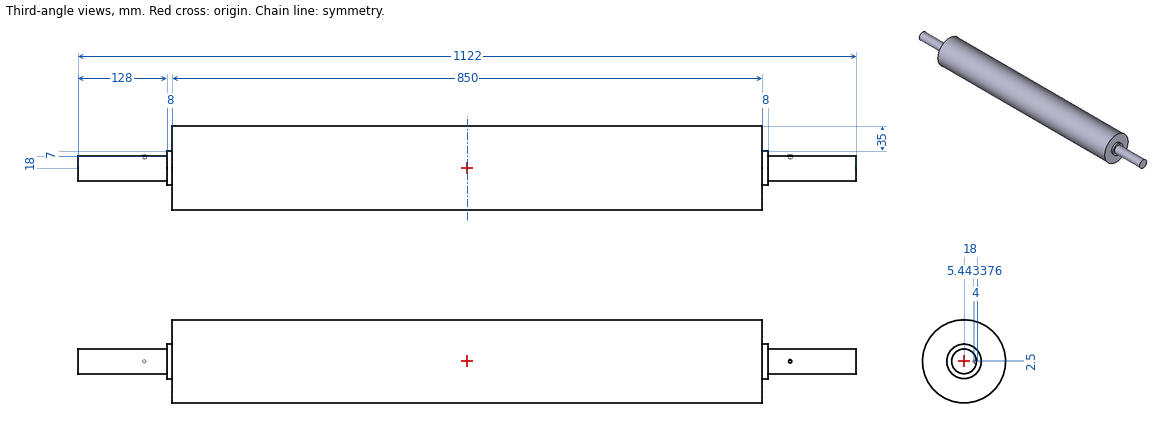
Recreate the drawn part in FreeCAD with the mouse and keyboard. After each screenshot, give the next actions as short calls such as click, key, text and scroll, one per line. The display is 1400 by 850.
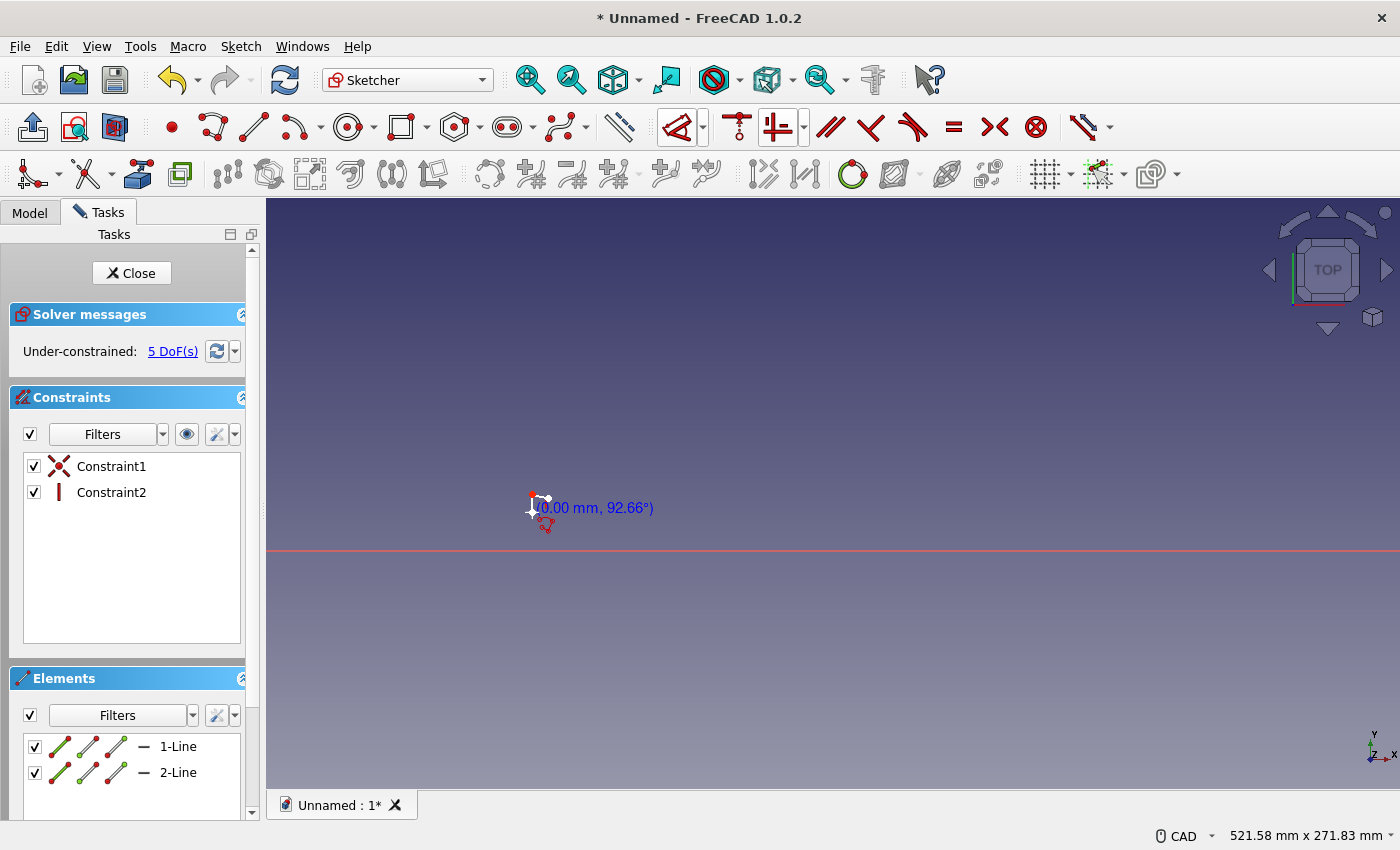
scroll(532, 496, down, 7)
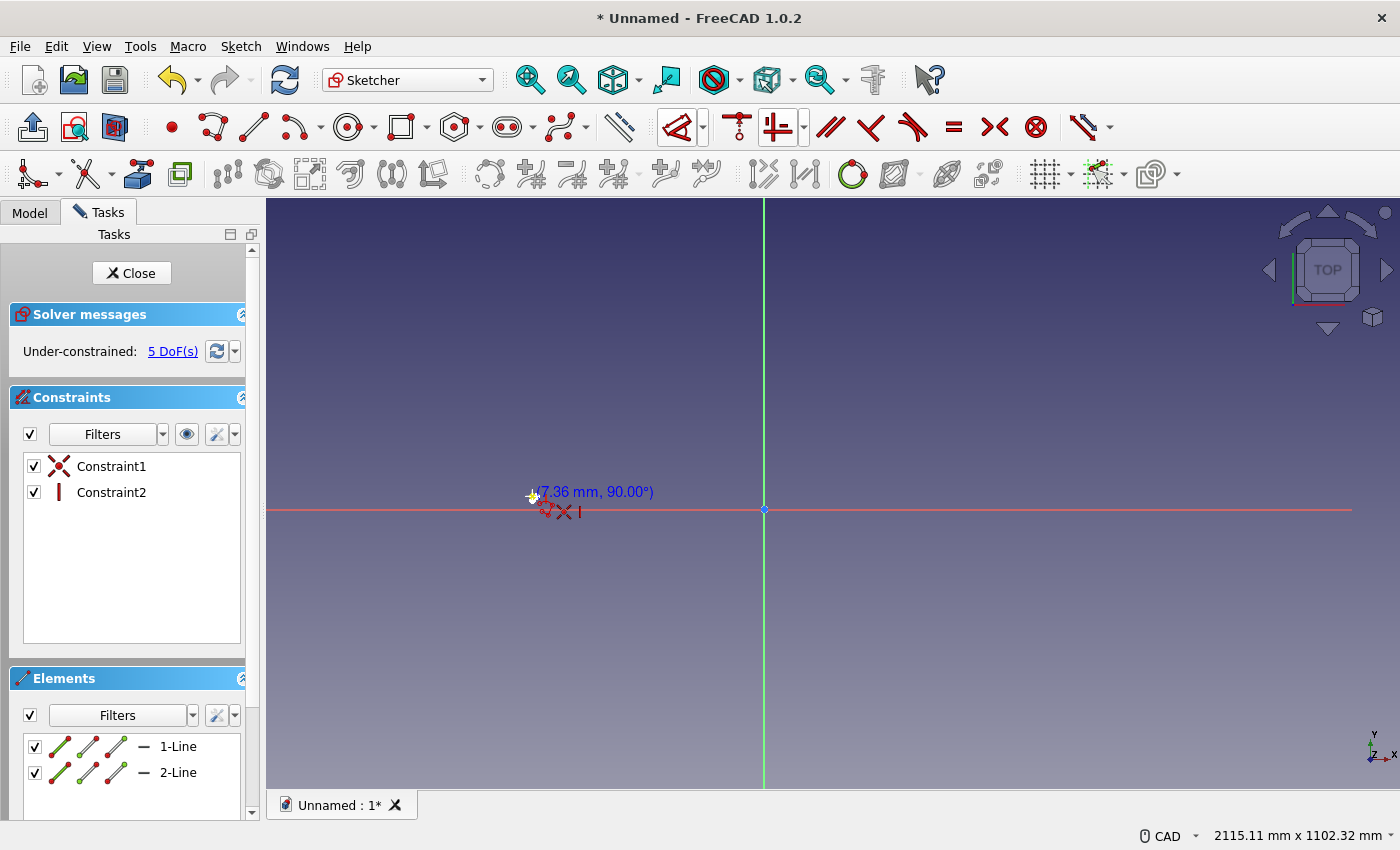
scroll(464, 500, up, 3)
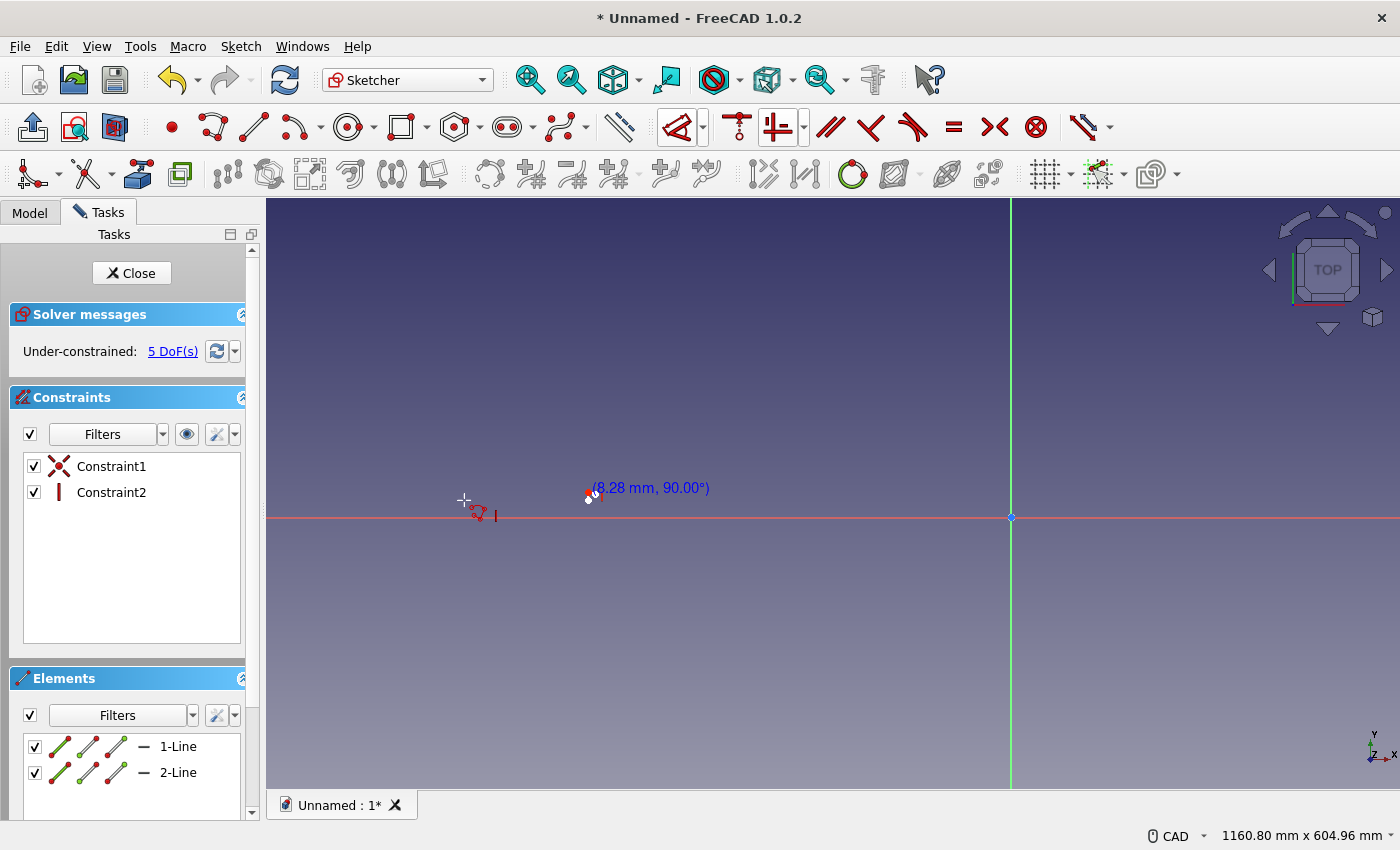
click(463, 500)
click(463, 518)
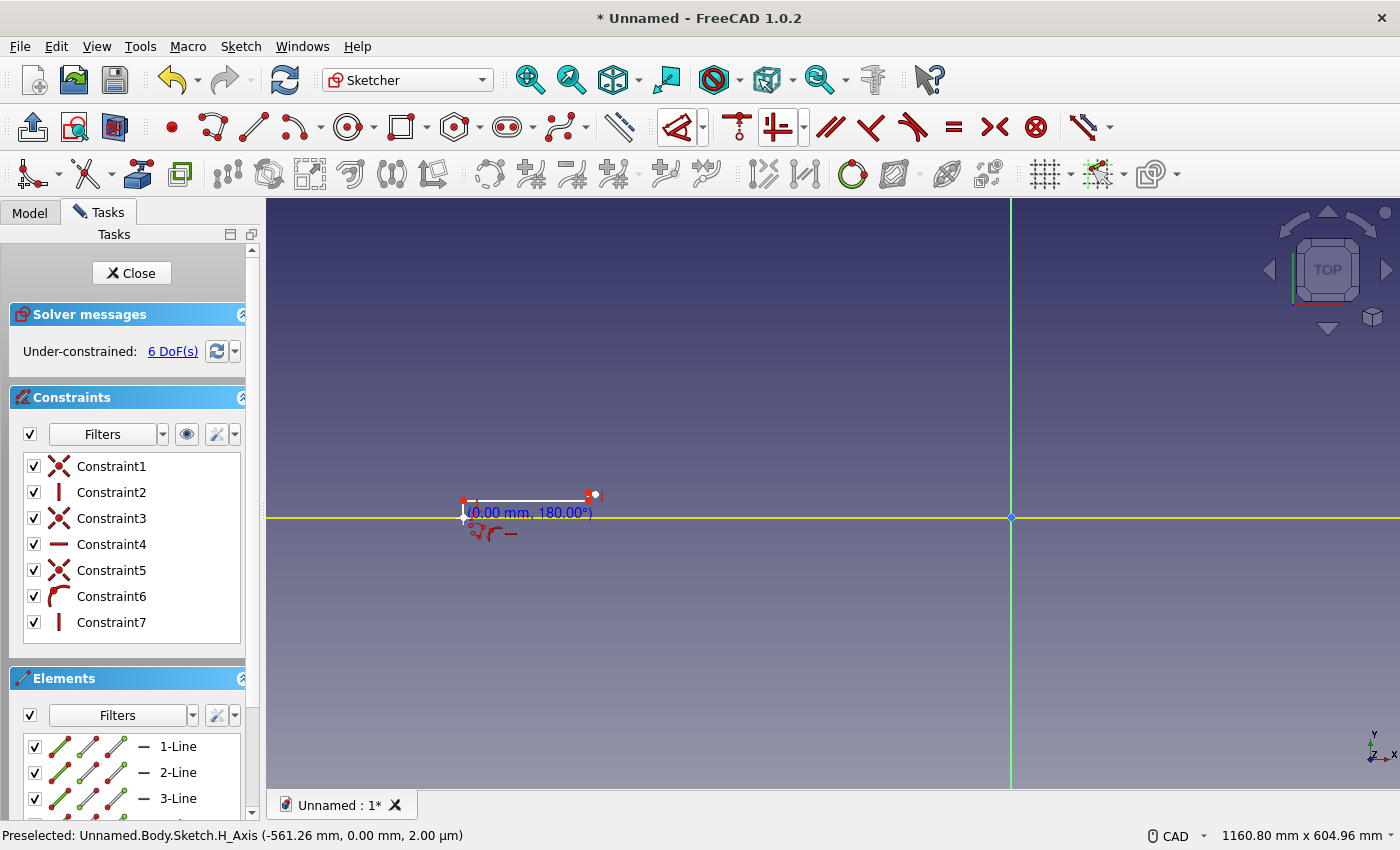
scroll(464, 500, down, 3)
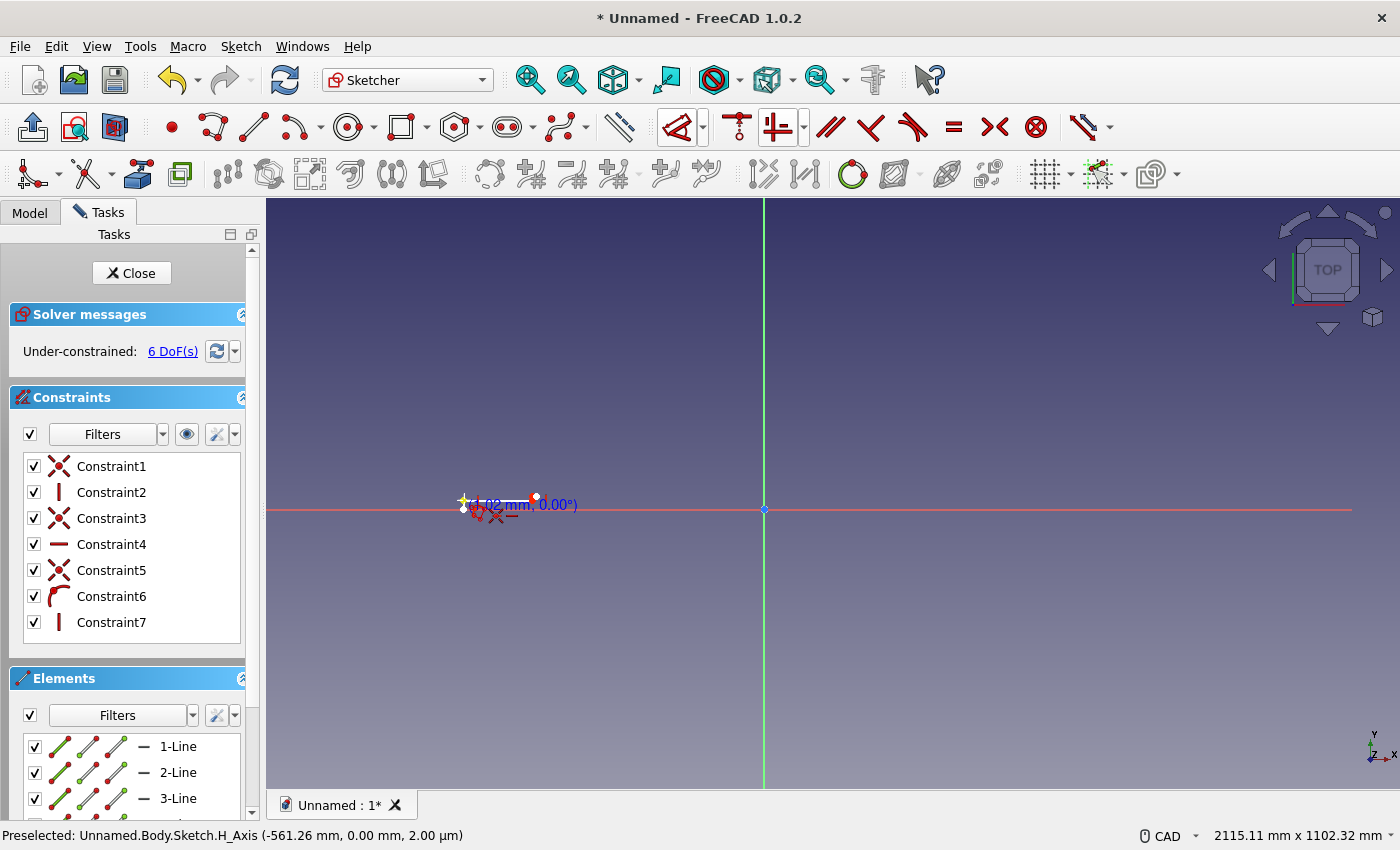
click(1065, 501)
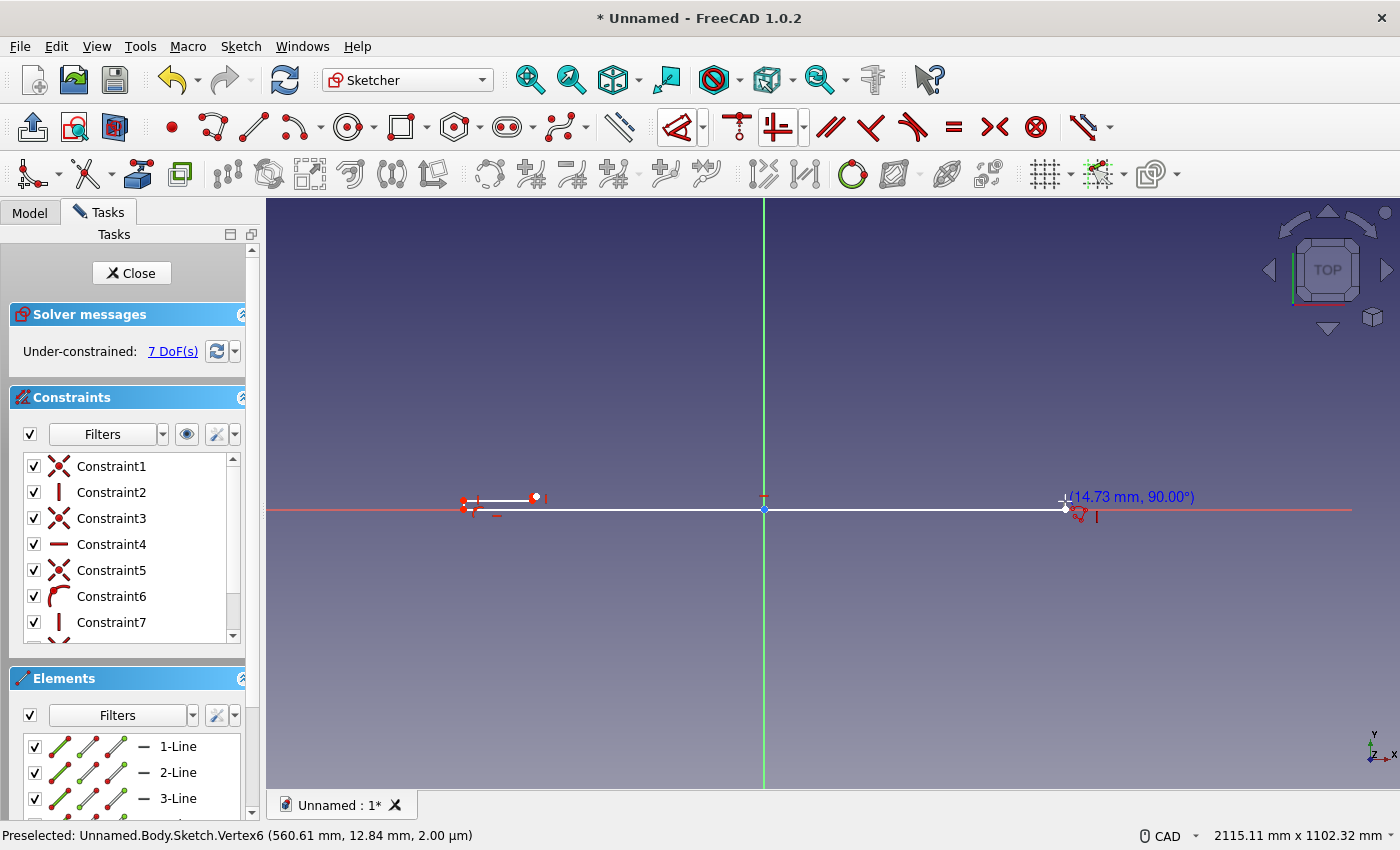
scroll(1065, 500, up, 3)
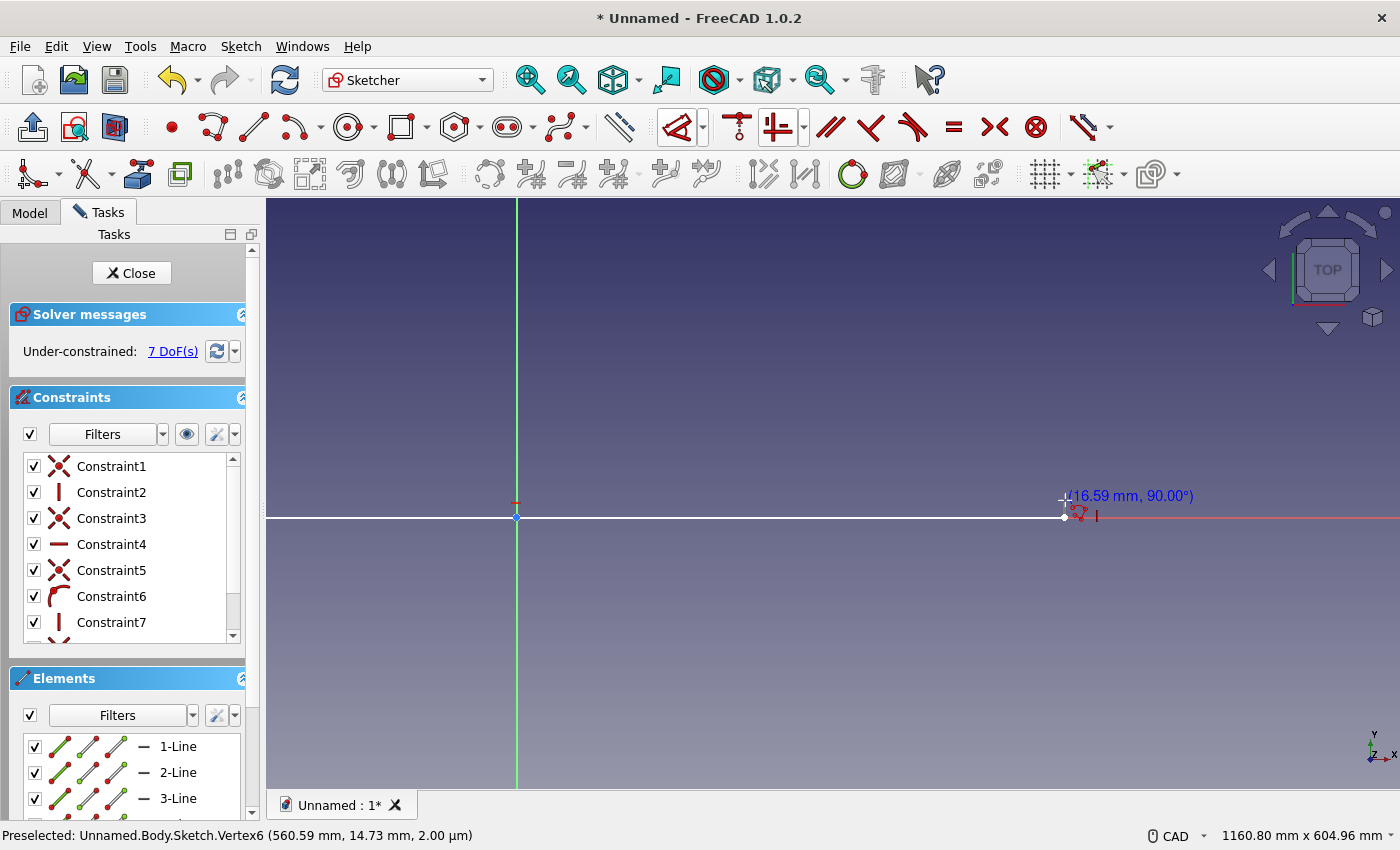
click(1064, 500)
click(940, 500)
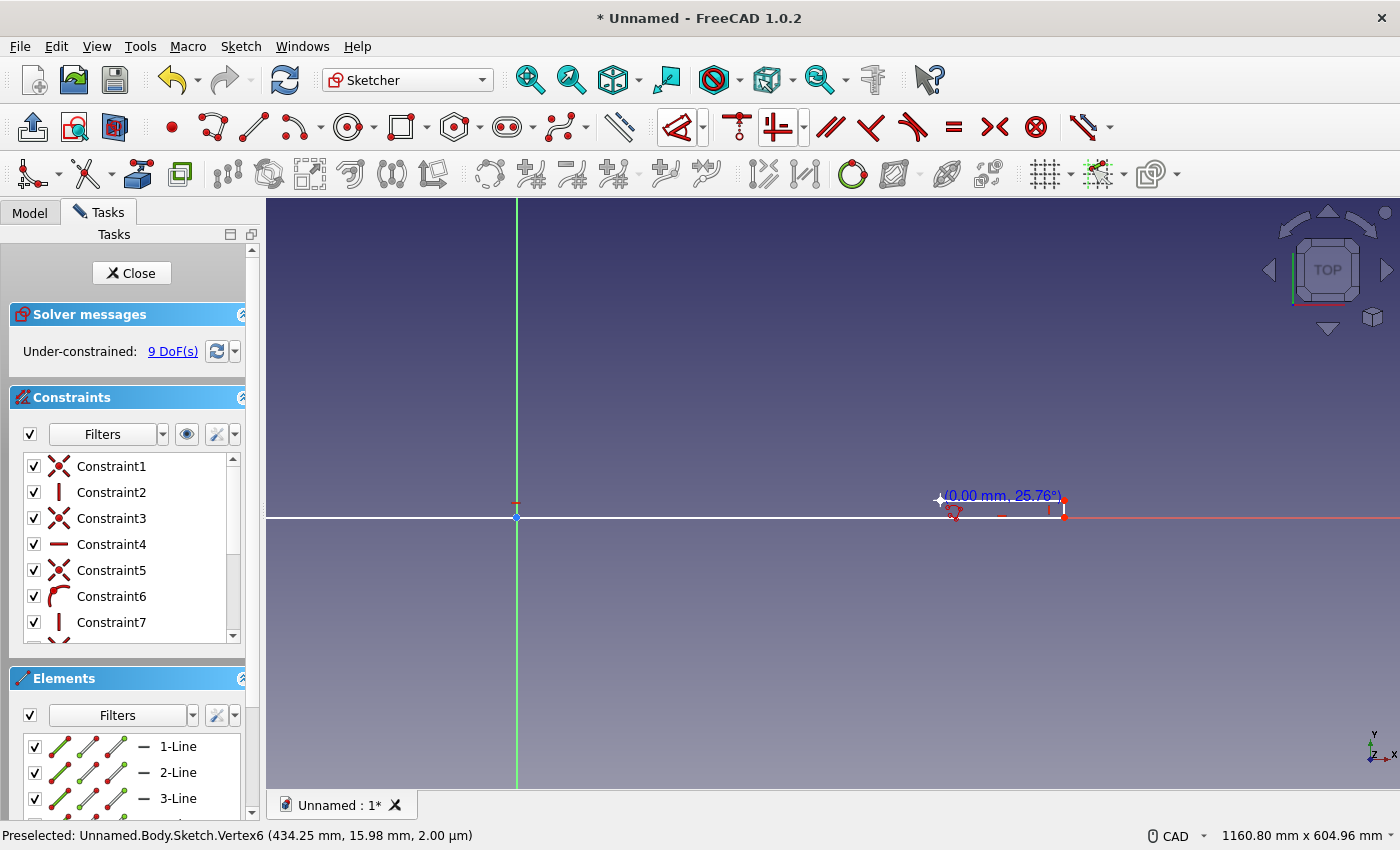
scroll(940, 493, up, 5)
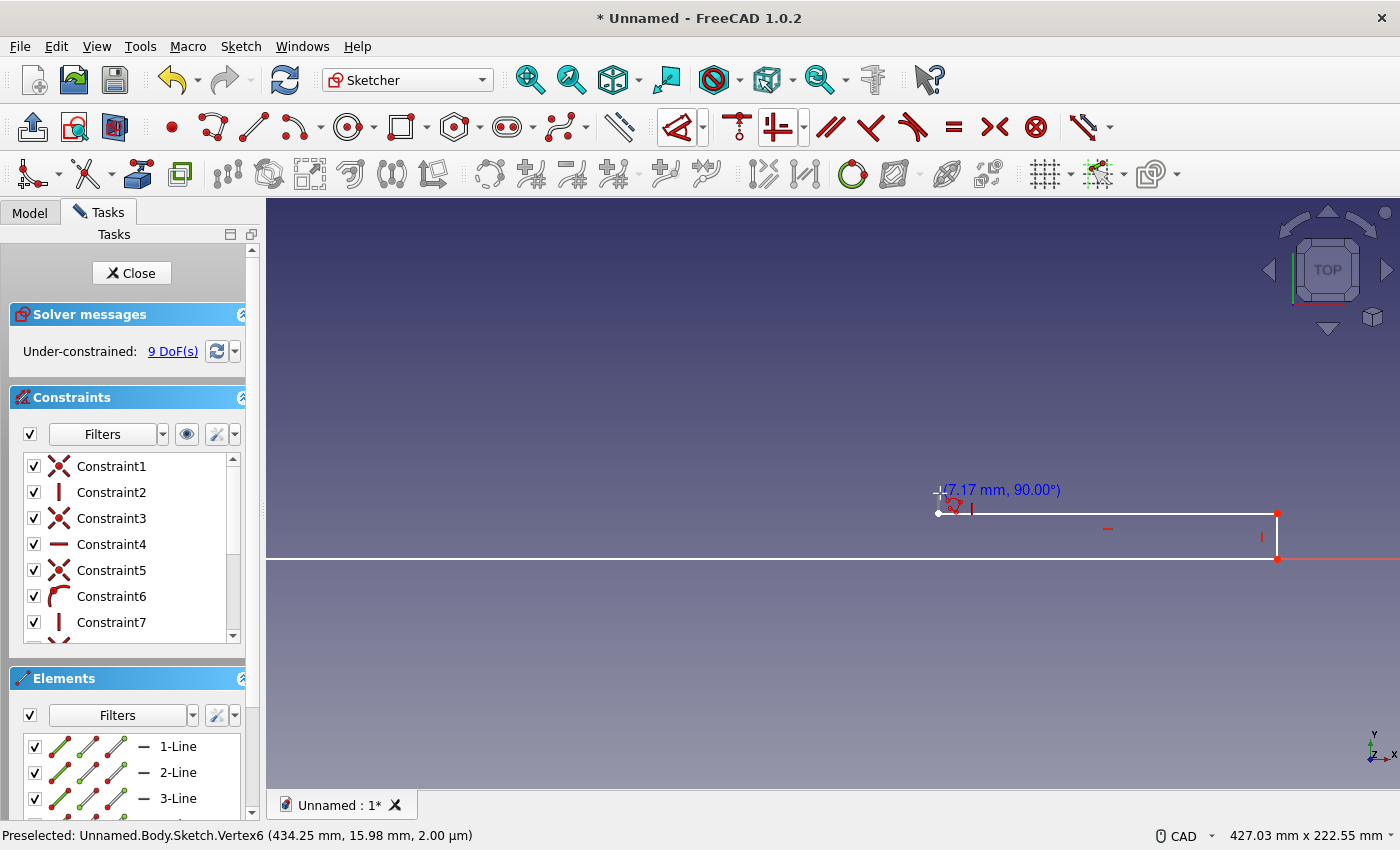
click(939, 493)
click(917, 493)